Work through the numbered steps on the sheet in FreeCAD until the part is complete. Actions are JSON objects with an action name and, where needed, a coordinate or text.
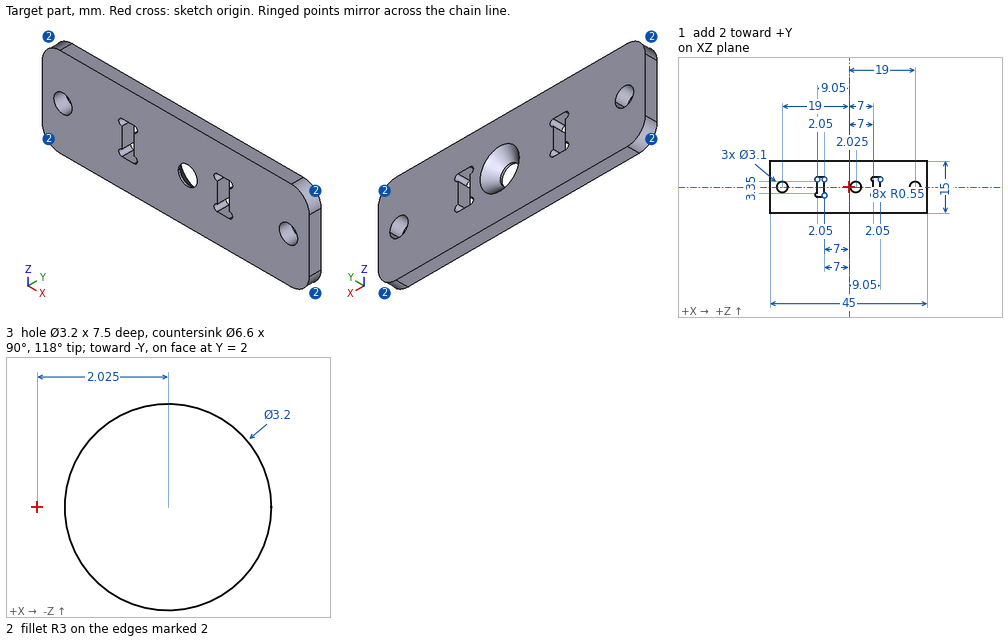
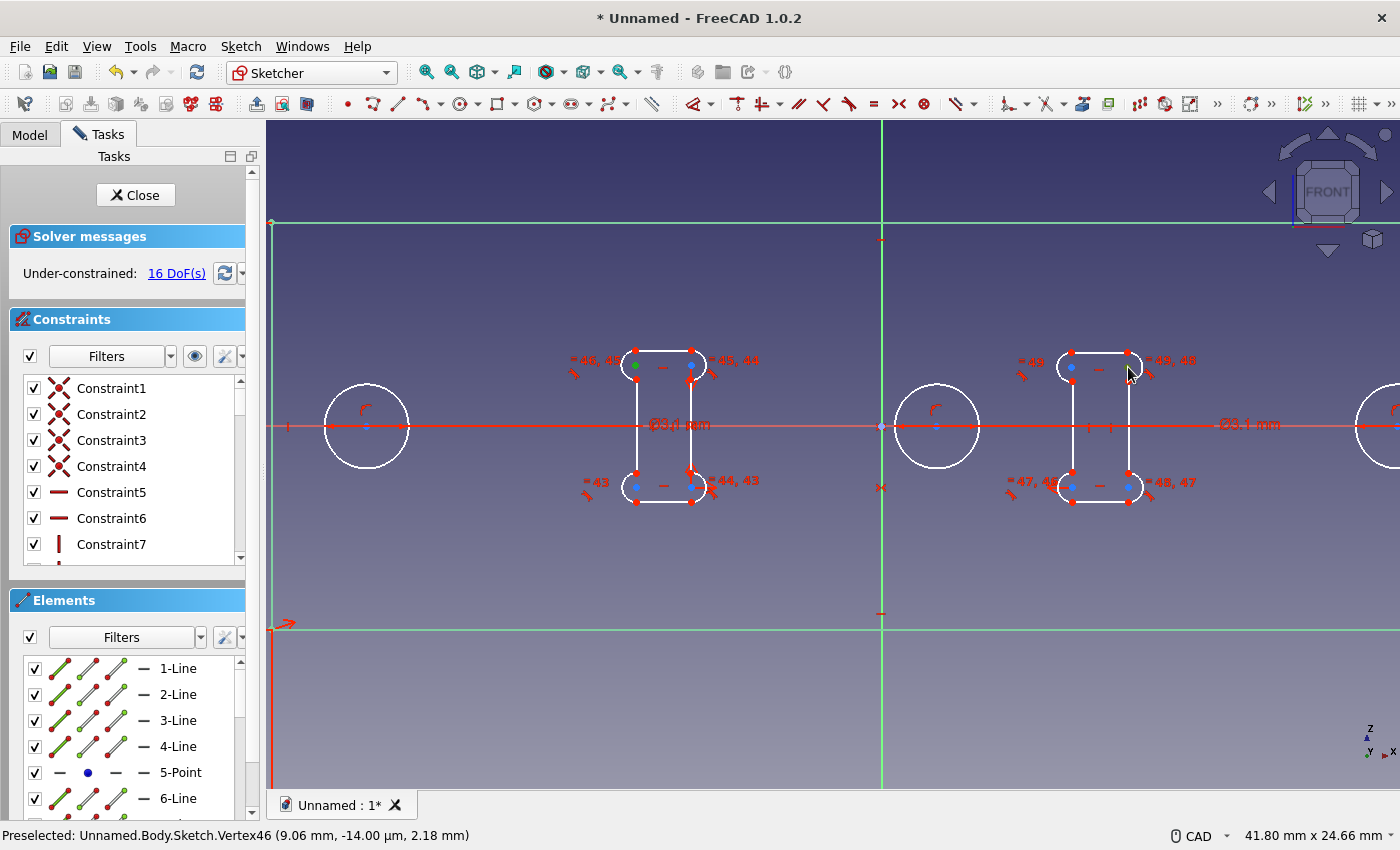
{"action": "left_click", "coordinate": [882, 717]}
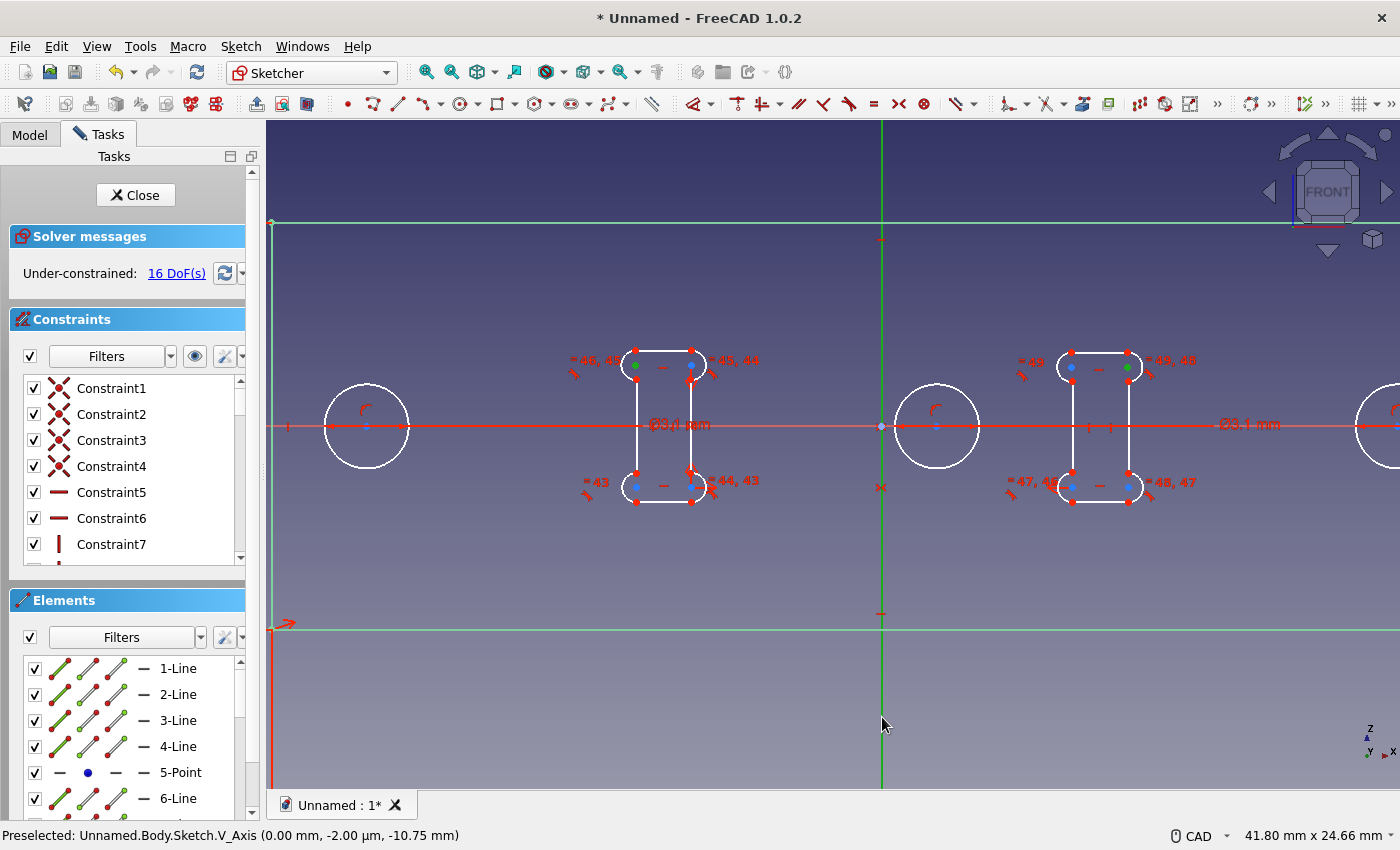
{"action": "left_click", "coordinate": [899, 104]}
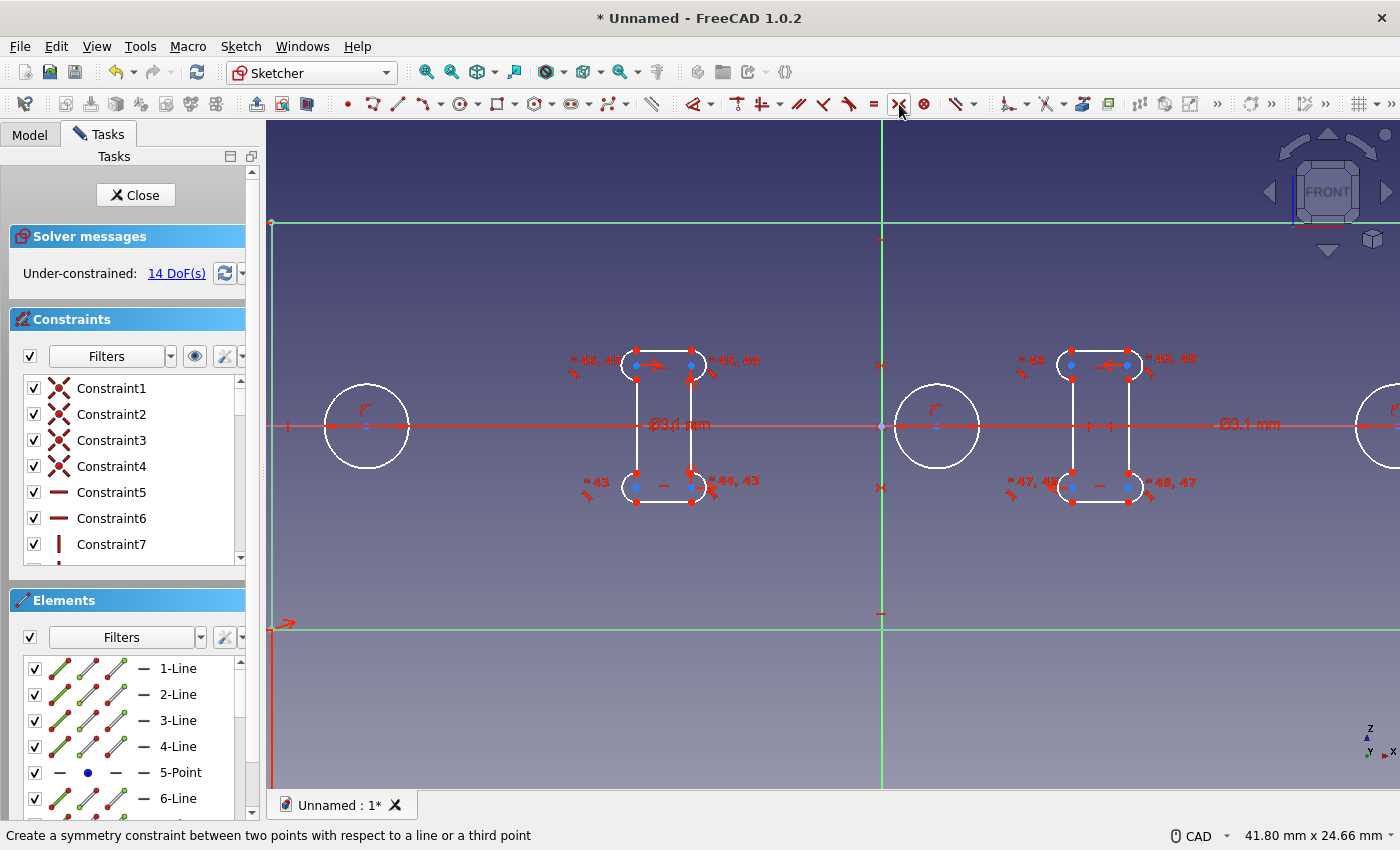
{"action": "left_click", "coordinate": [692, 104]}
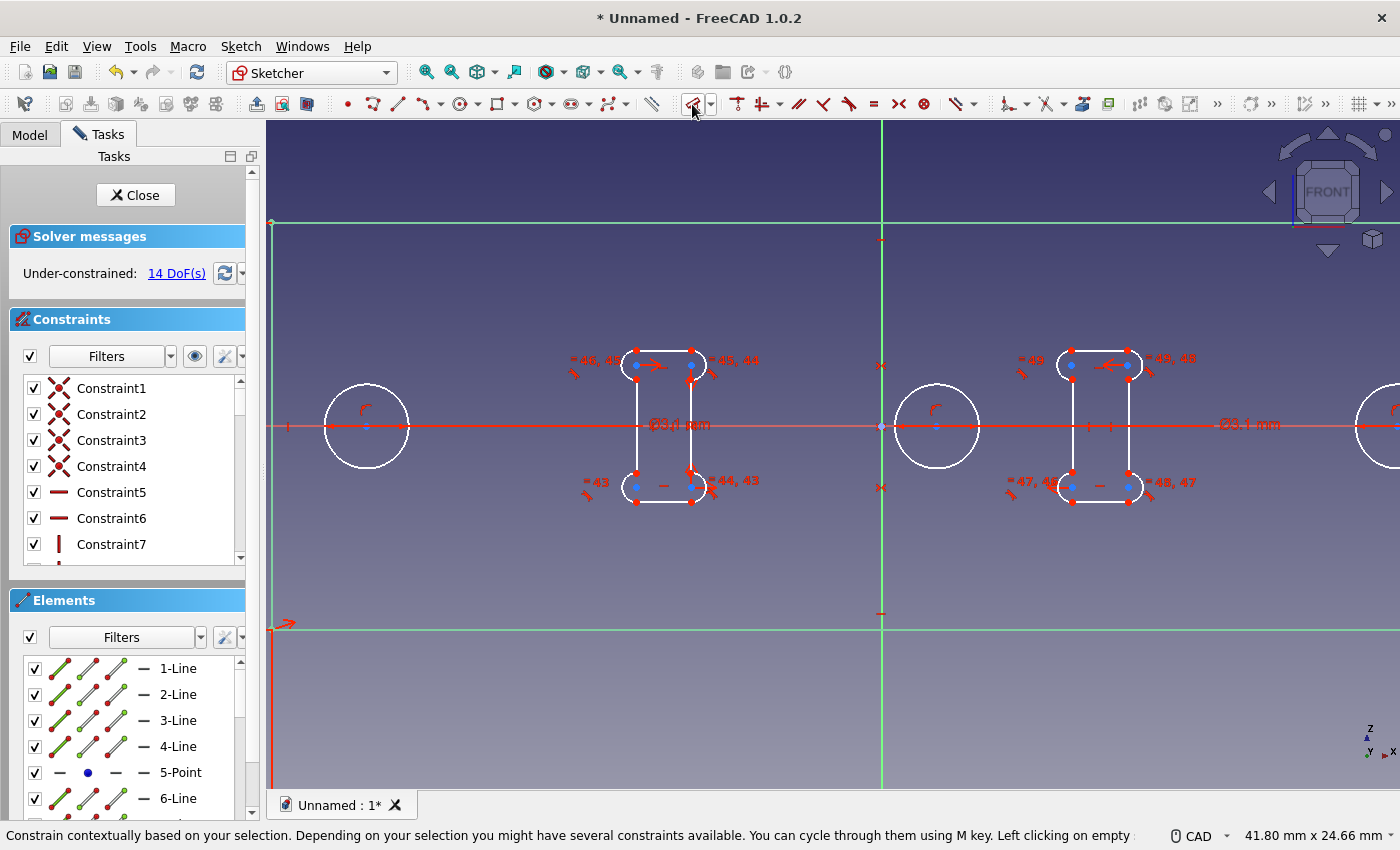
{"action": "scroll", "coordinate": [625, 479], "scroll_direction": "up", "scroll_amount": 5}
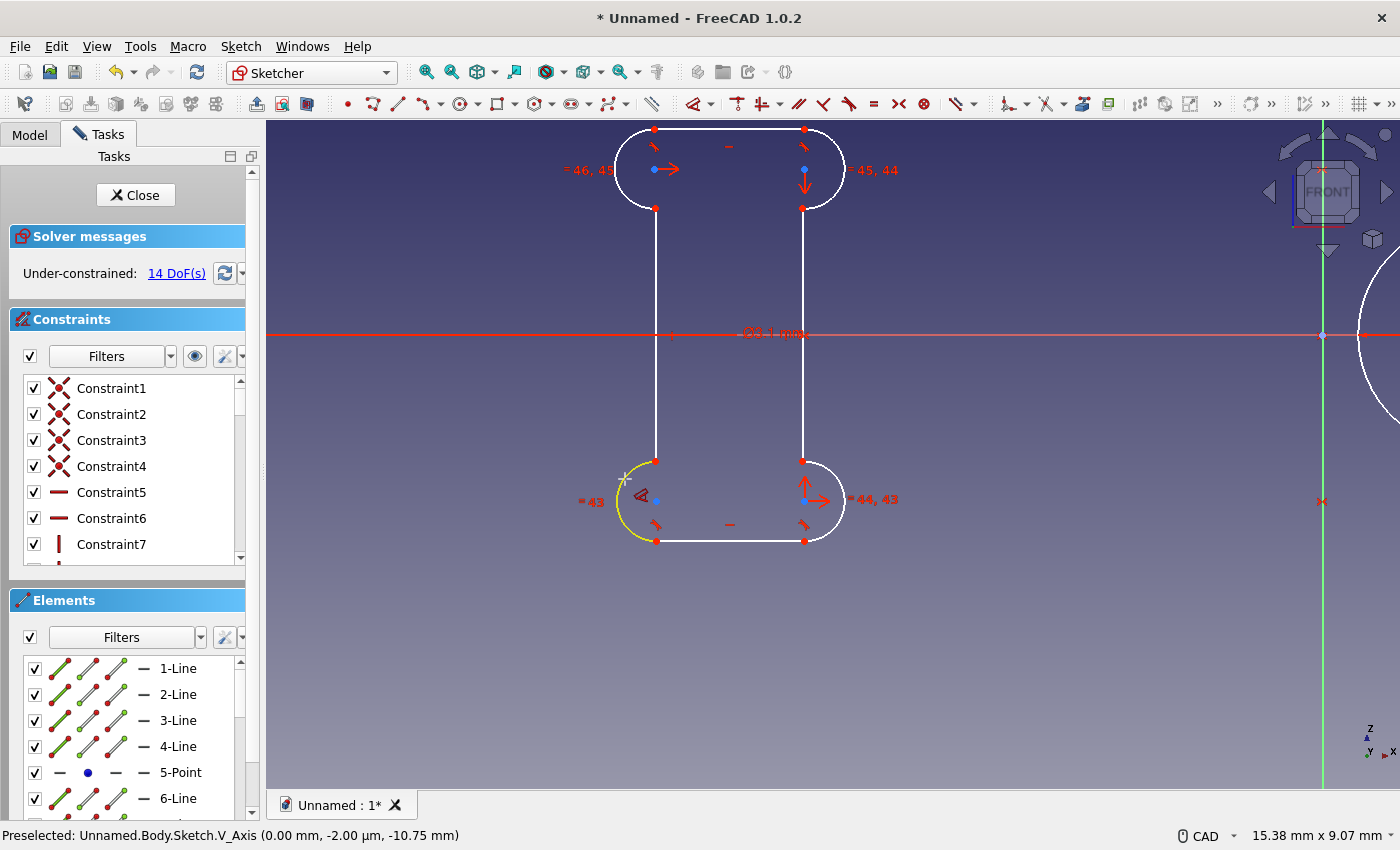
{"action": "left_click", "coordinate": [624, 479]}
{"action": "left_click", "coordinate": [598, 461]}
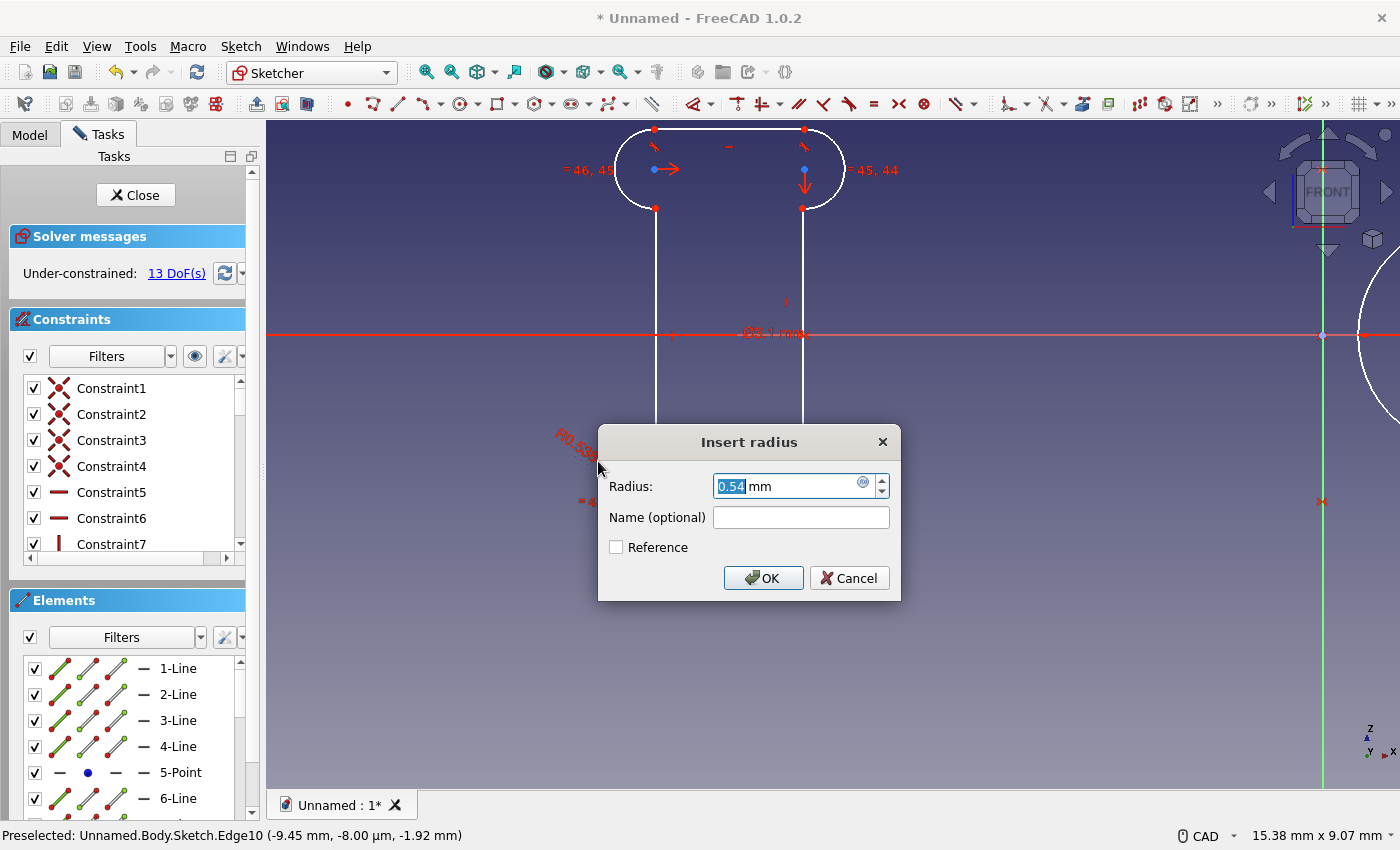
{"action": "type", "text": "0.55"}
{"action": "key", "text": "Return"}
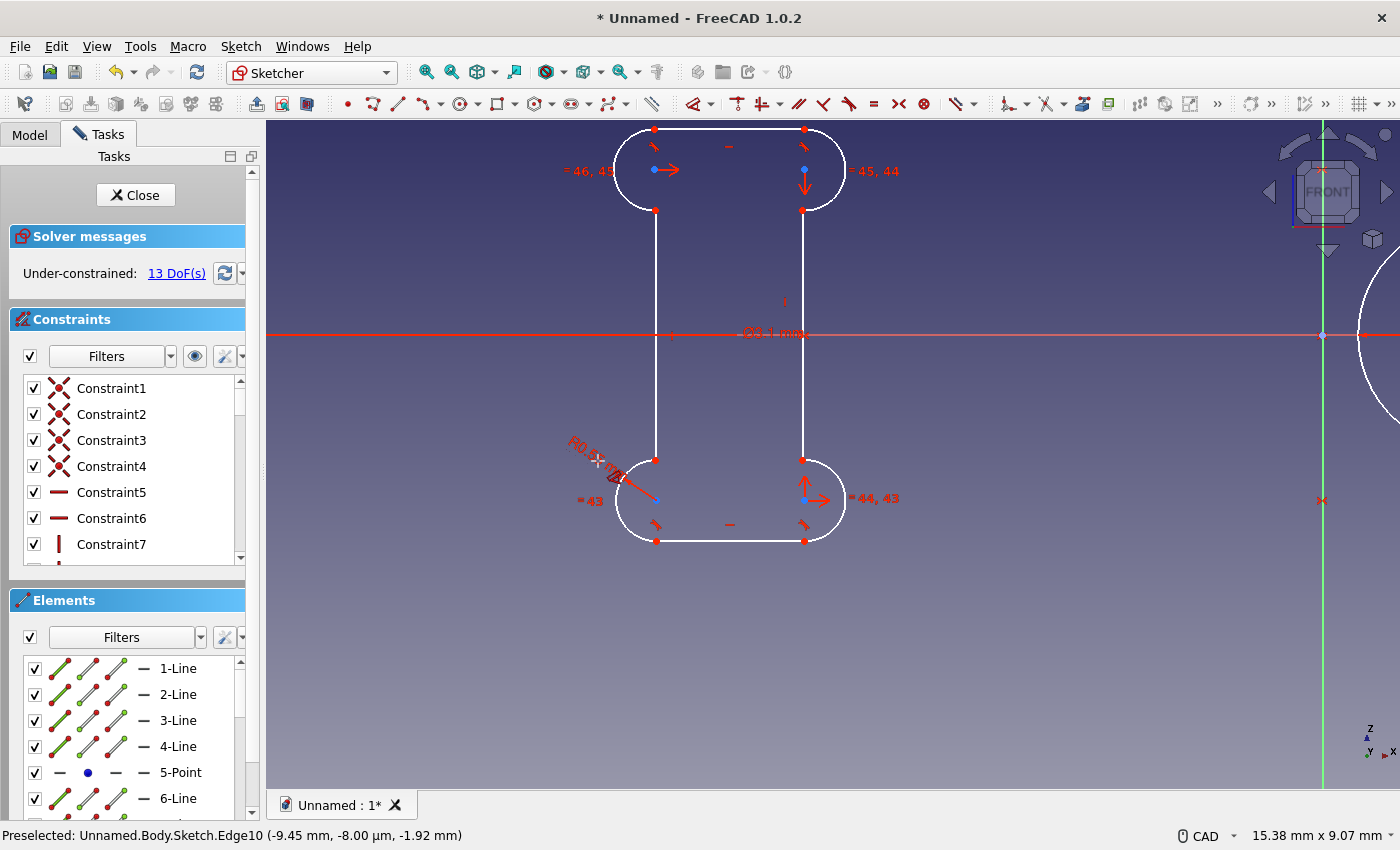
{"action": "scroll", "coordinate": [623, 485], "scroll_direction": "down", "scroll_amount": 8}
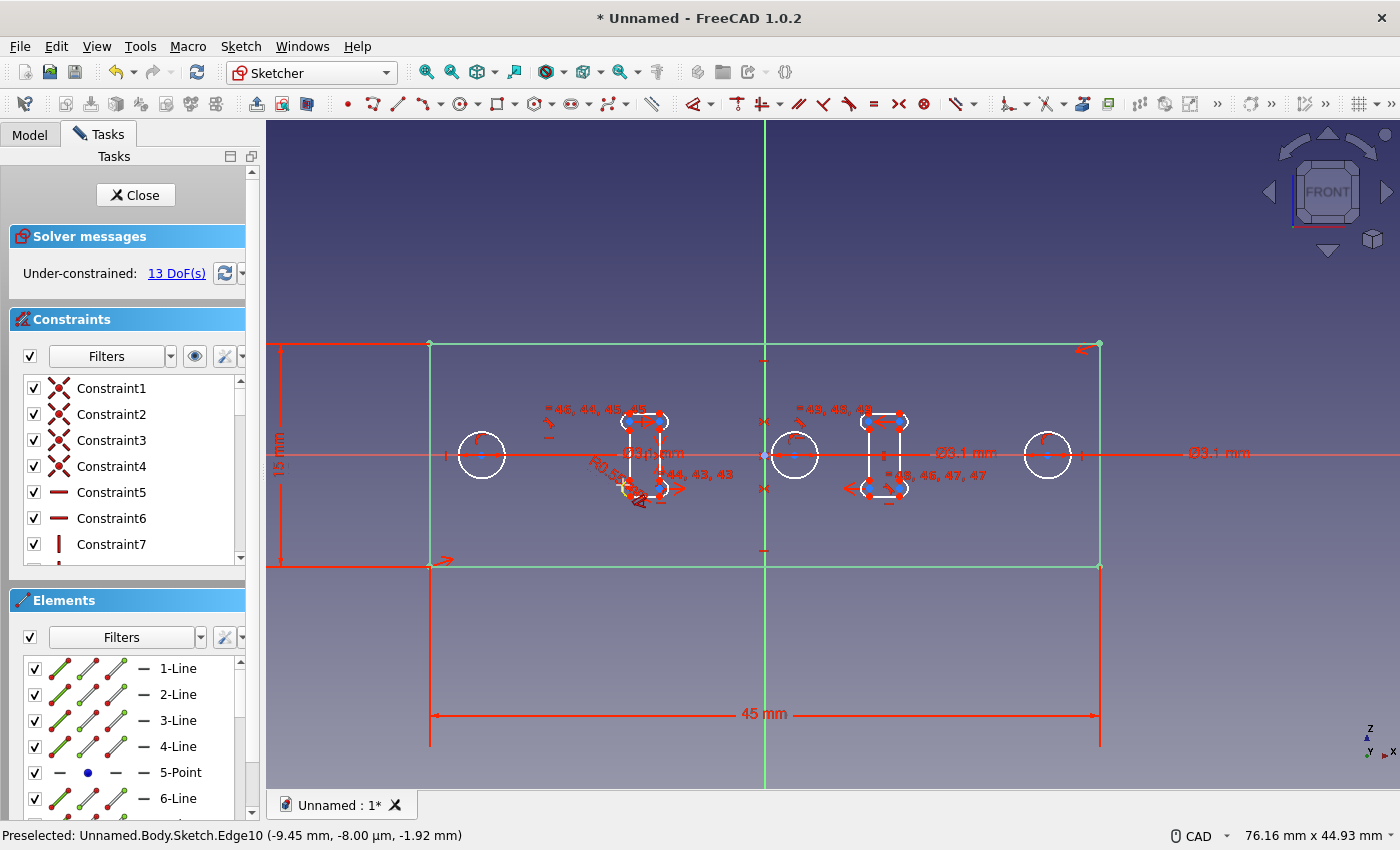
{"action": "scroll", "coordinate": [660, 497], "scroll_direction": "up", "scroll_amount": 2}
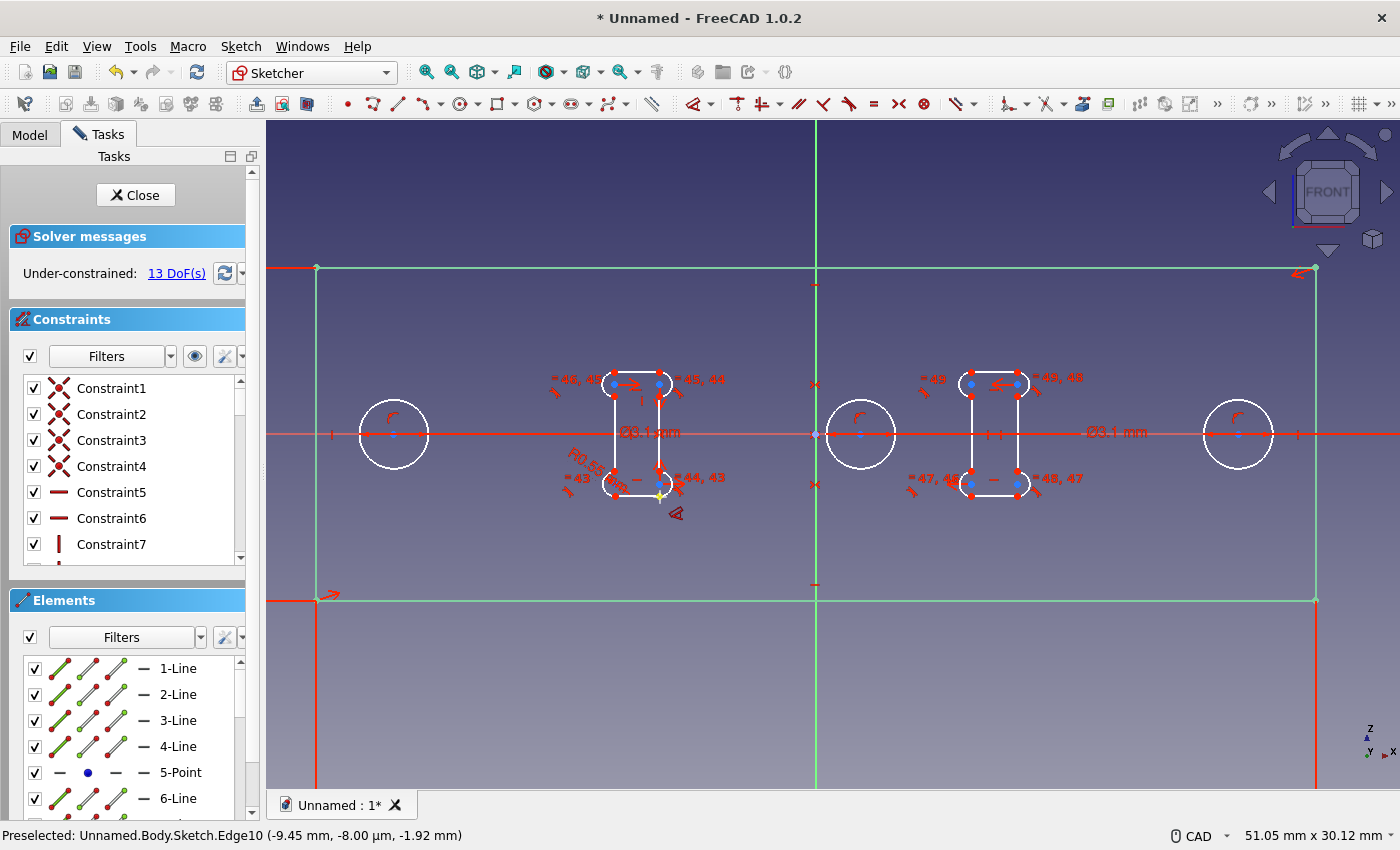
{"action": "left_click", "coordinate": [660, 496]}
{"action": "left_click", "coordinate": [738, 530]}